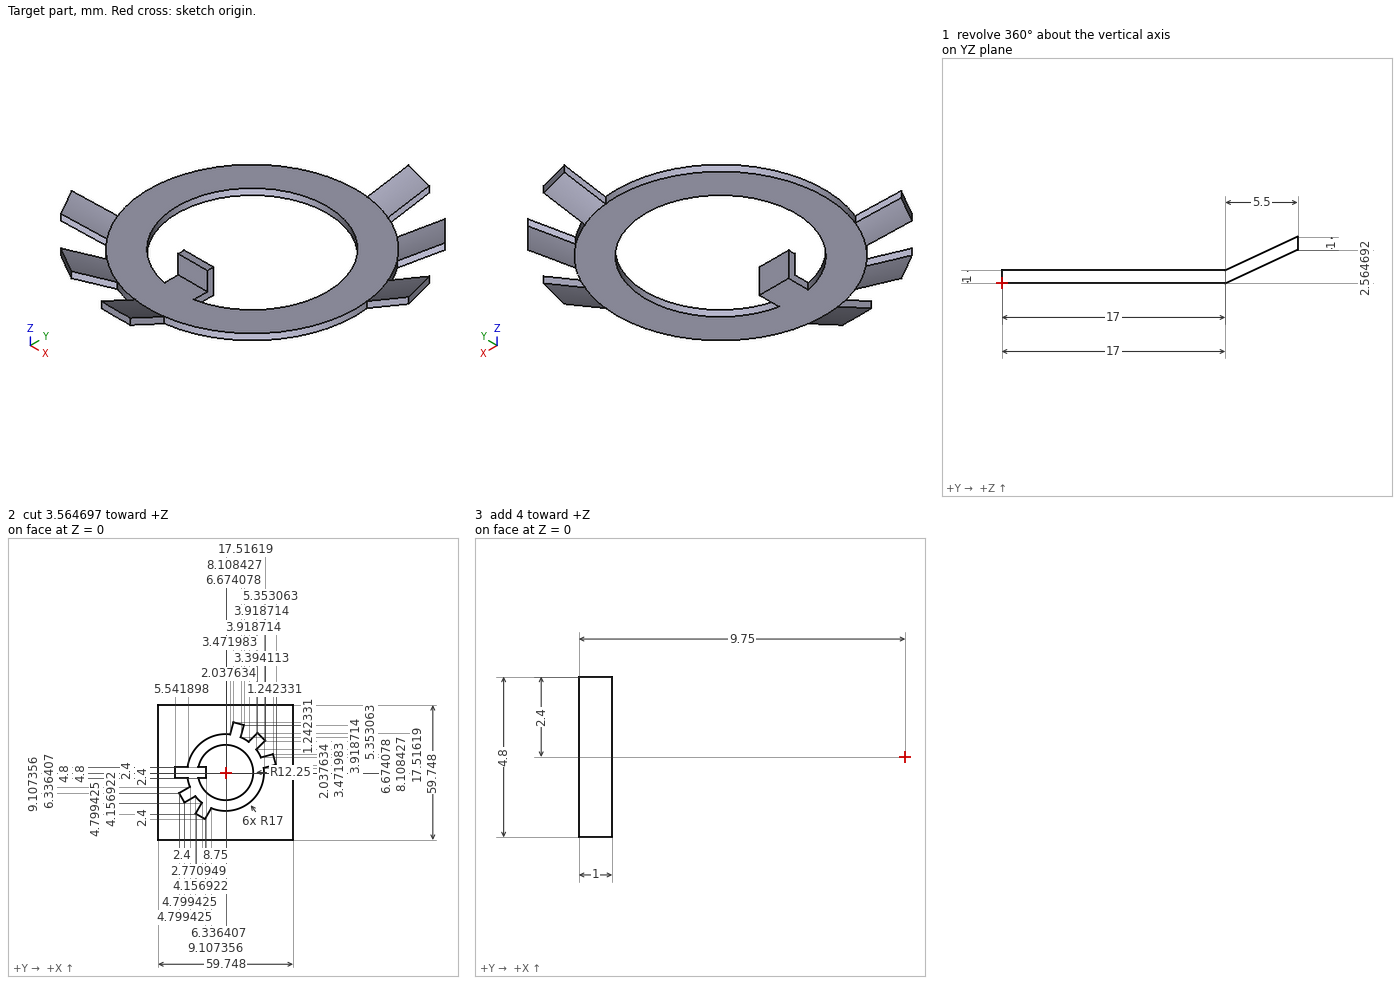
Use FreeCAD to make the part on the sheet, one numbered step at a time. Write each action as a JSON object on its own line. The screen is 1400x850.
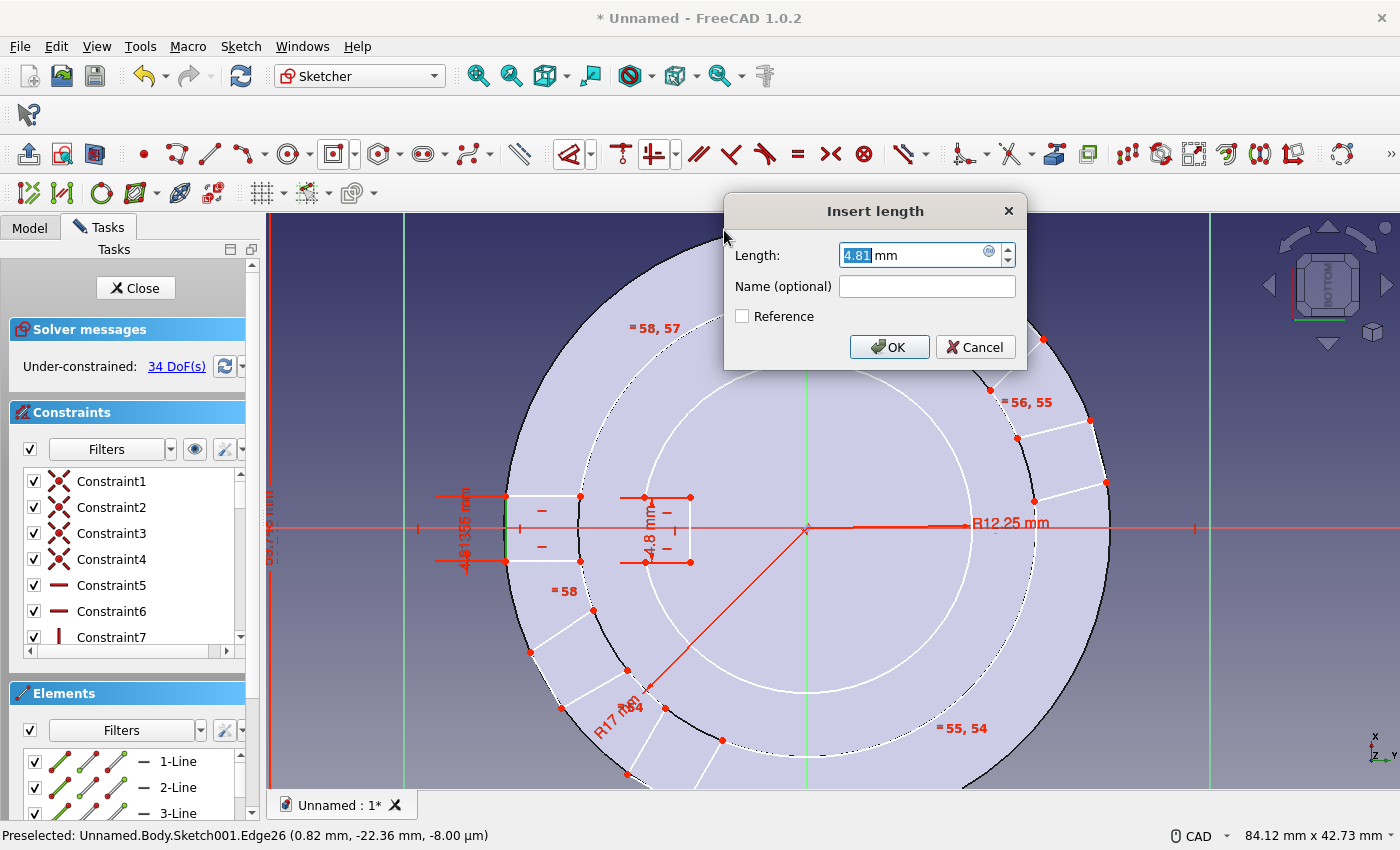
{"action": "type", "text": "4.8"}
{"action": "key", "text": "Return"}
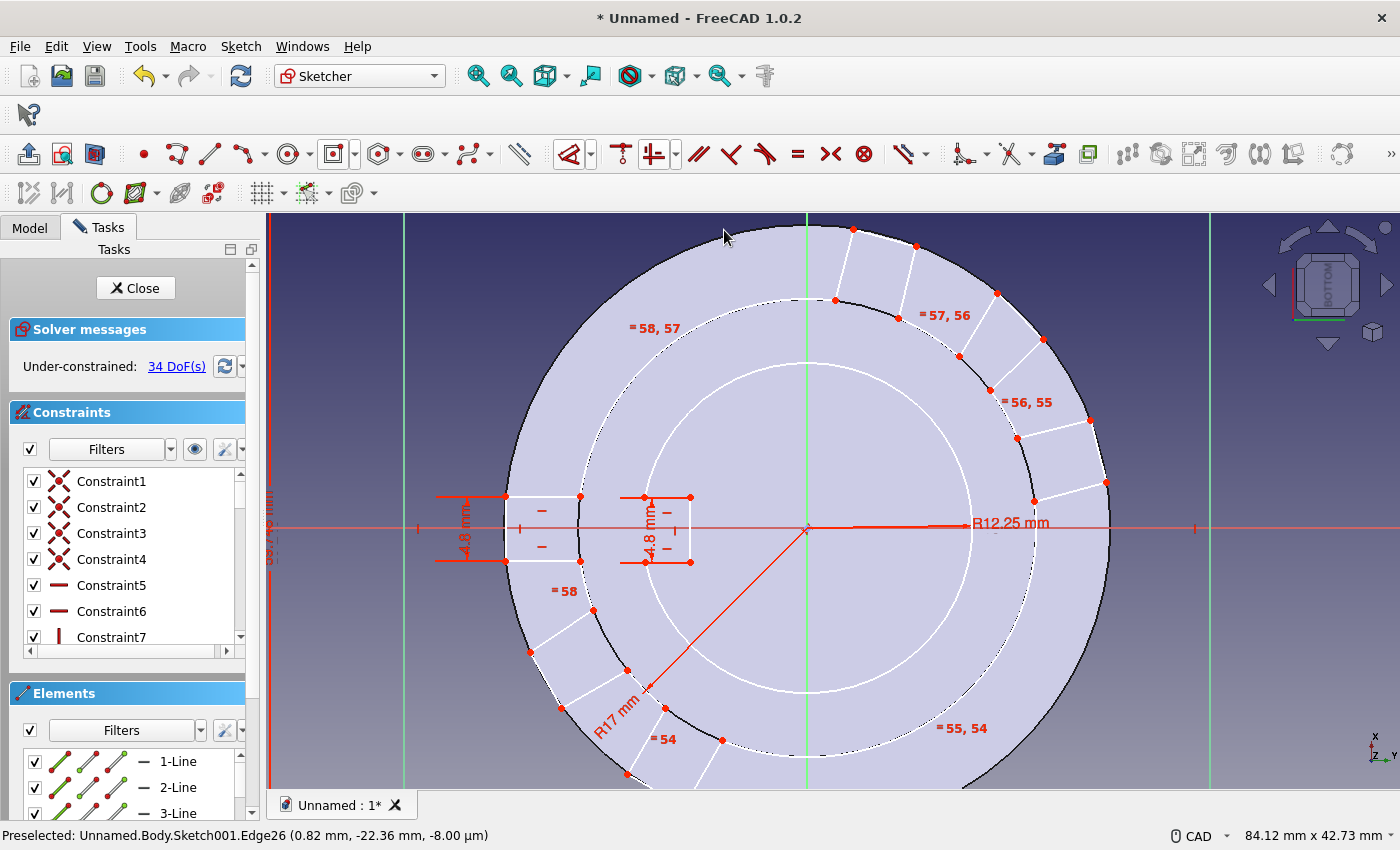
{"action": "scroll", "coordinate": [646, 563], "scroll_direction": "up", "scroll_amount": 2}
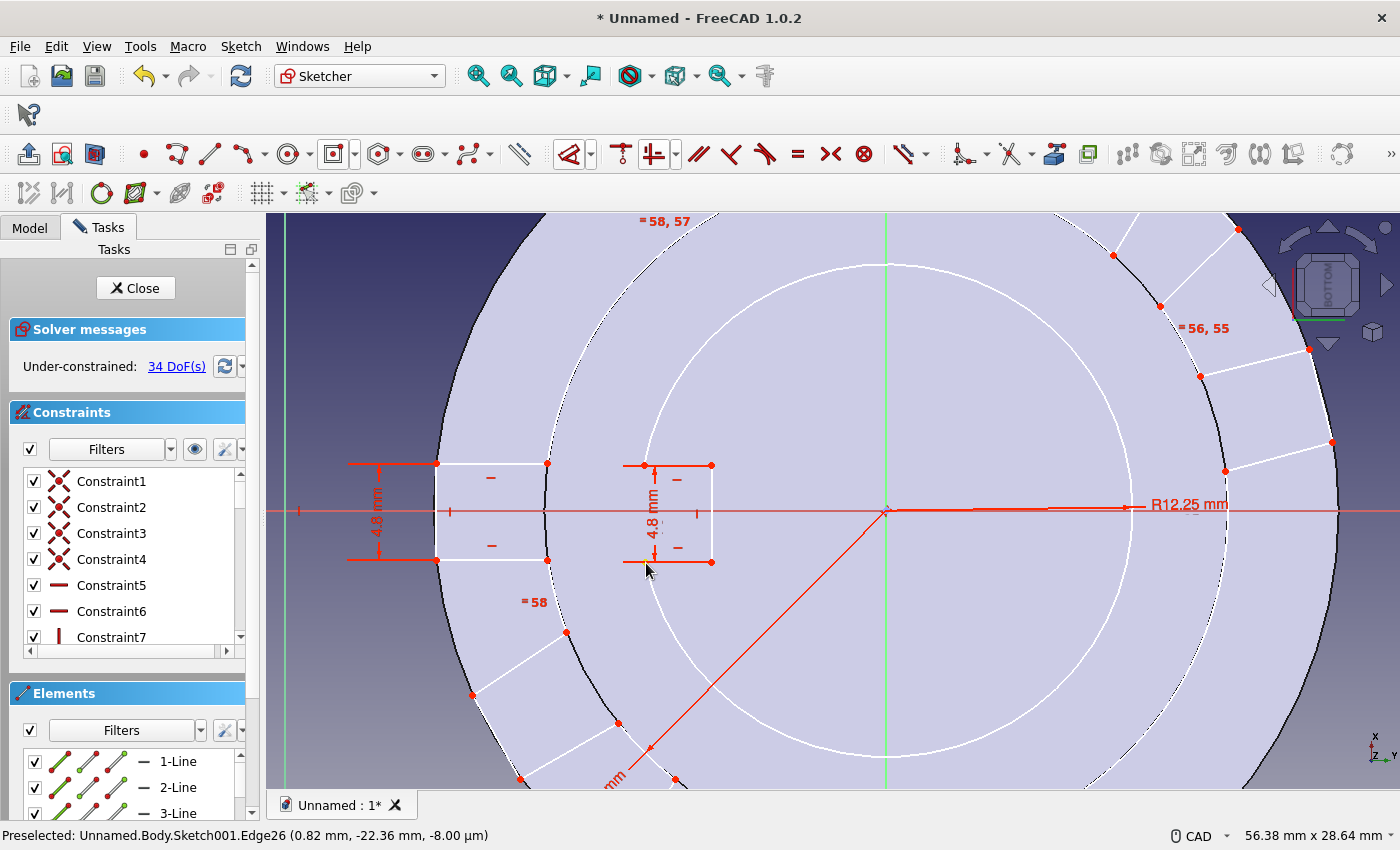
{"action": "left_click", "coordinate": [645, 562]}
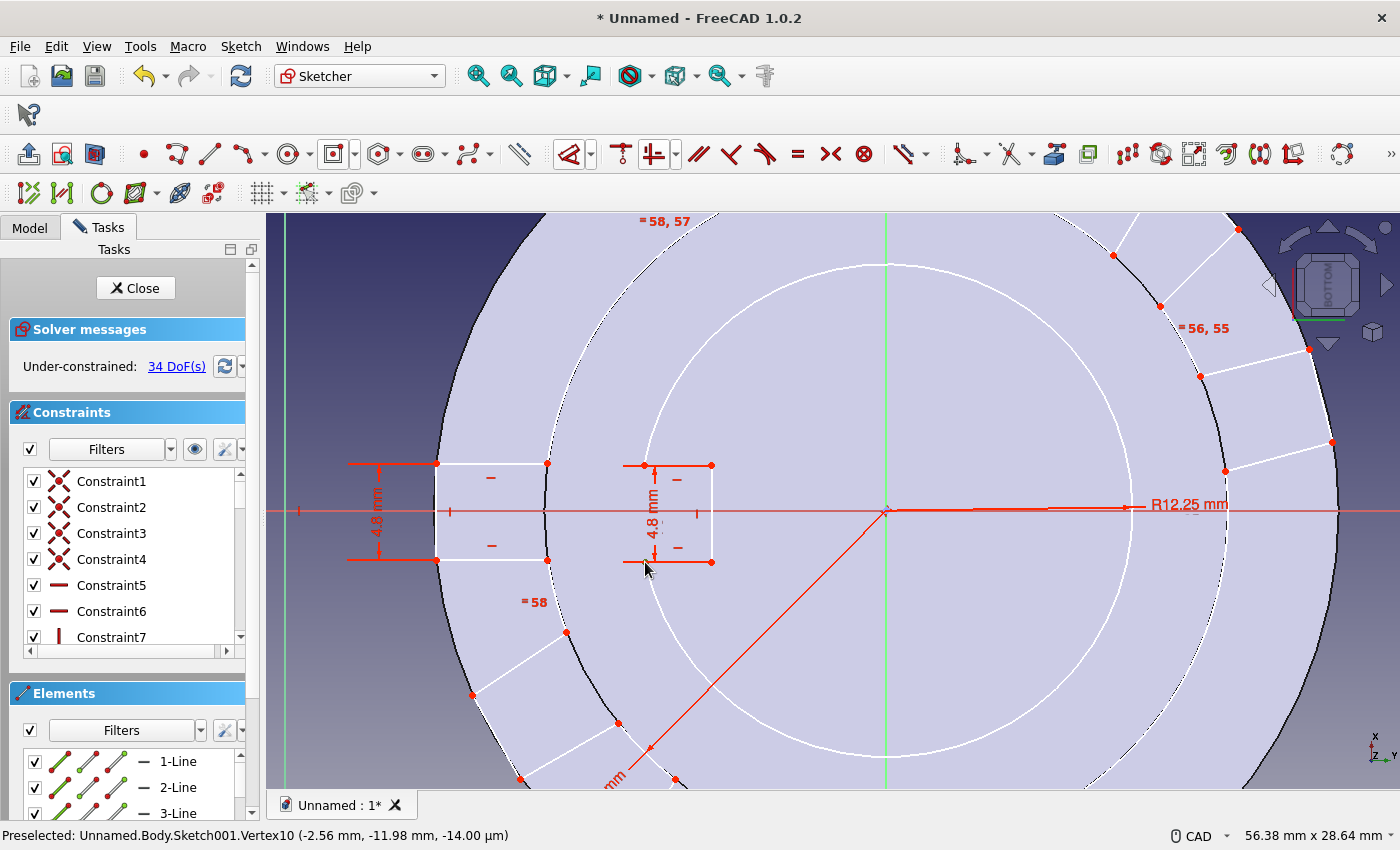
{"action": "key", "text": "i"}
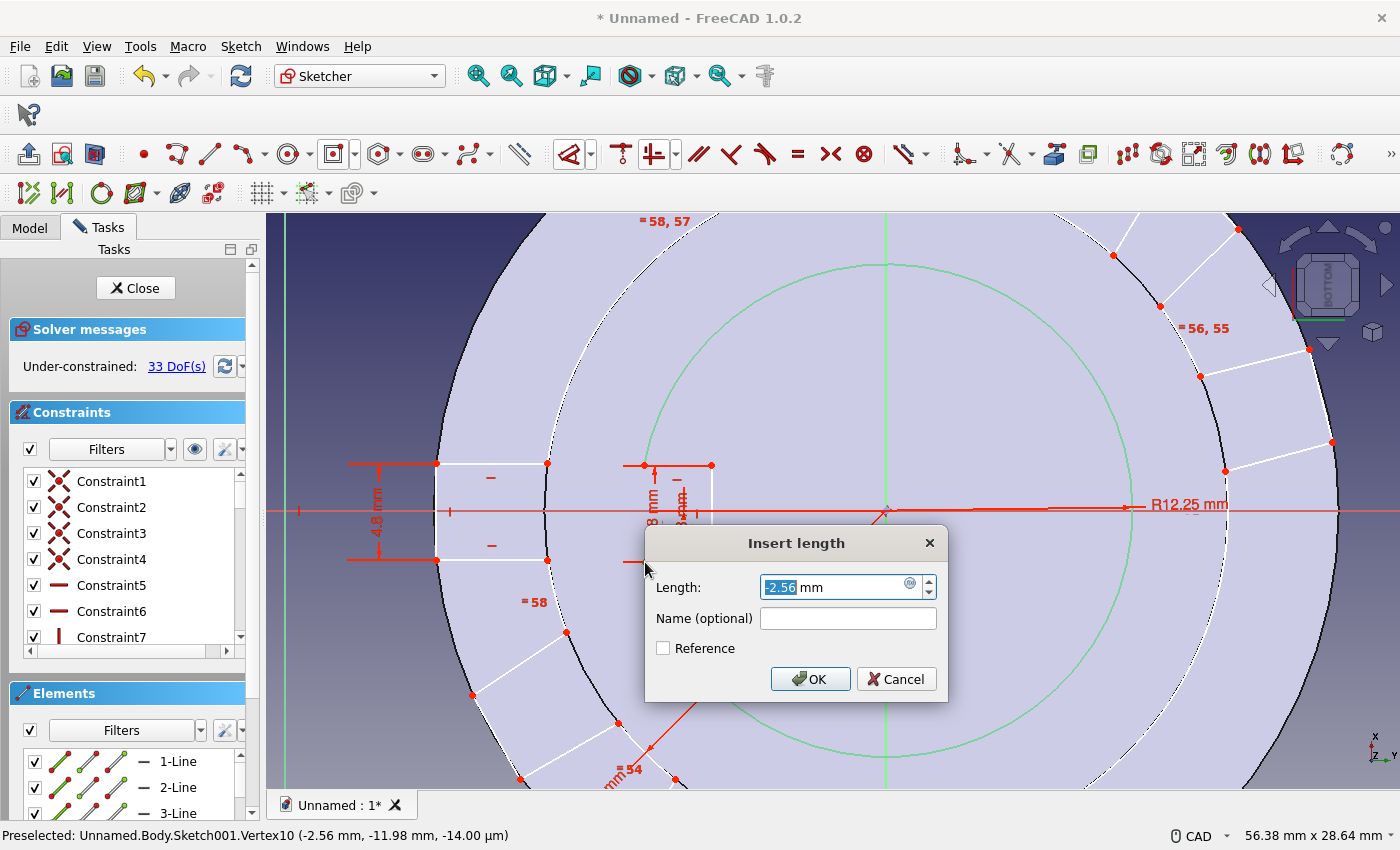
{"action": "type", "text": "-2.4"}
{"action": "key", "text": "Return"}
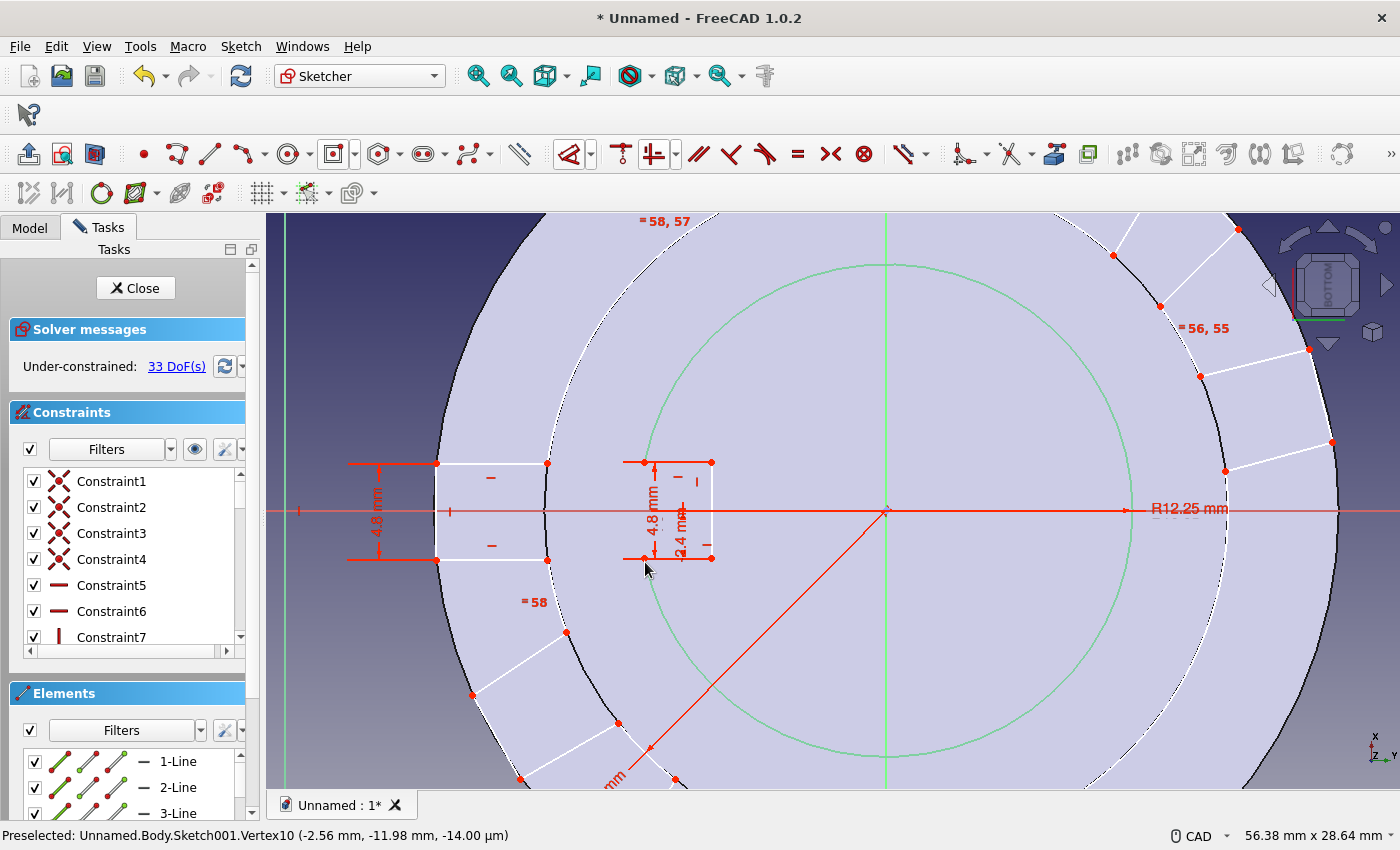
{"action": "left_click", "coordinate": [548, 464]}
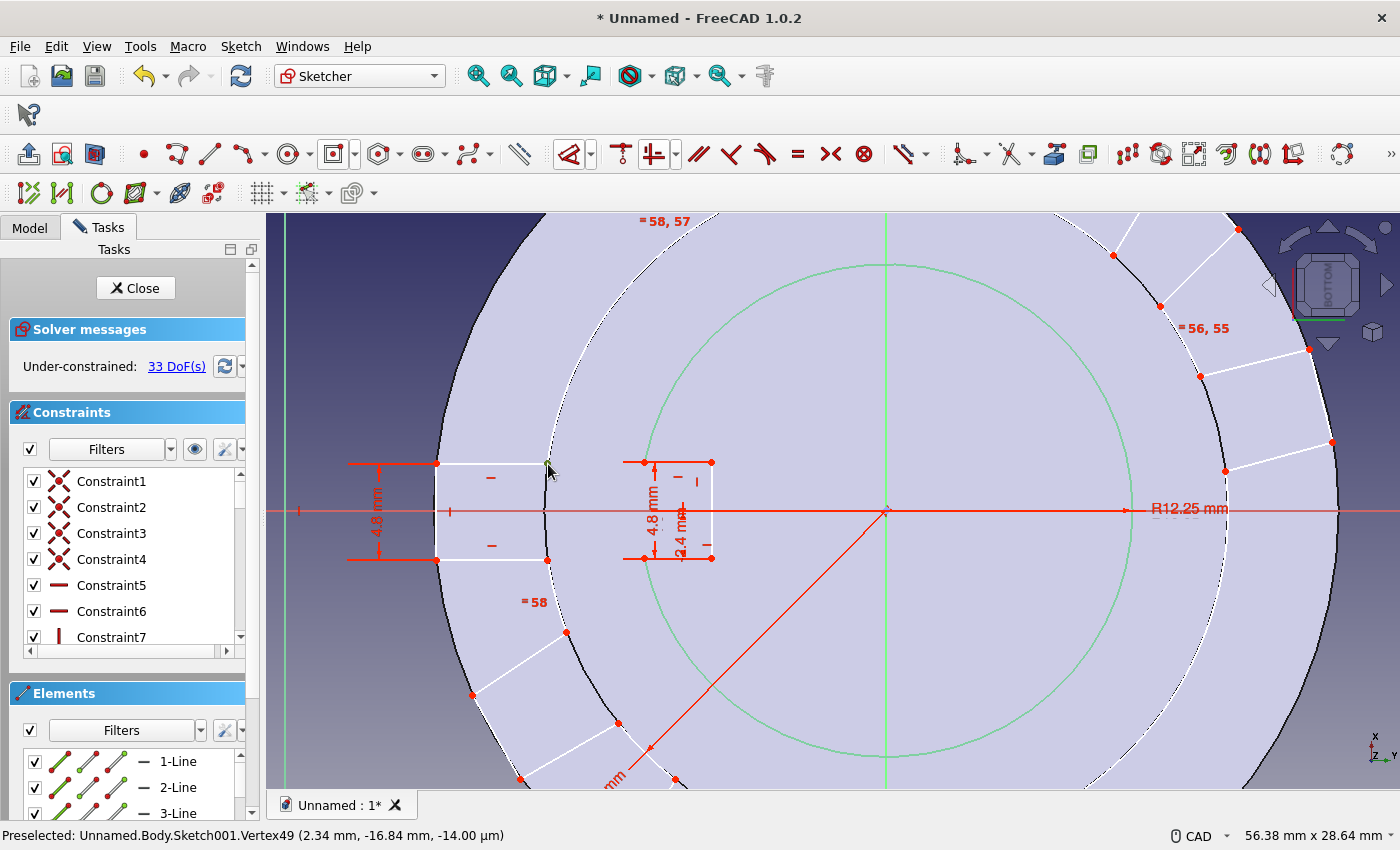
{"action": "left_click", "coordinate": [590, 154]}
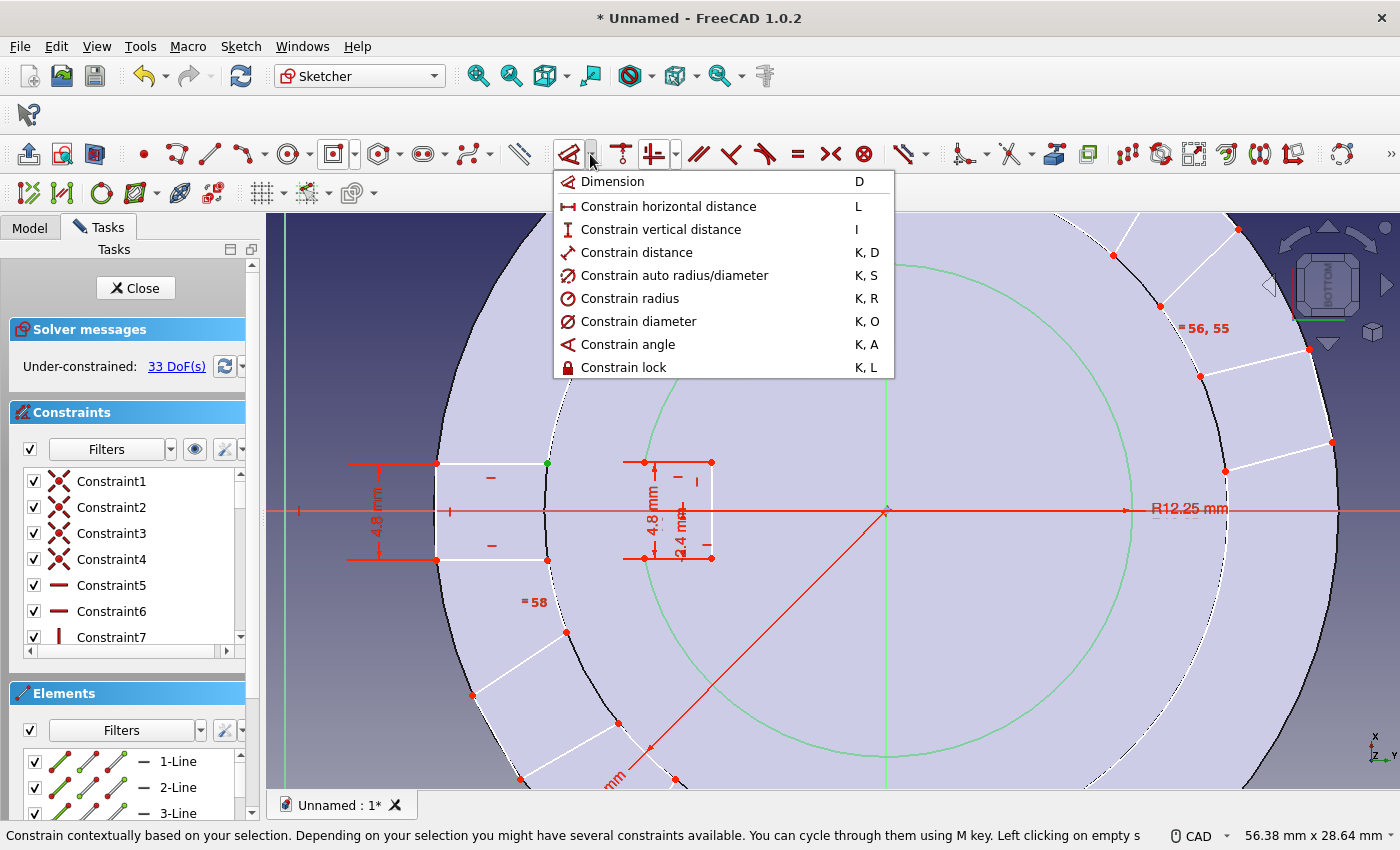
{"action": "left_click", "coordinate": [724, 230]}